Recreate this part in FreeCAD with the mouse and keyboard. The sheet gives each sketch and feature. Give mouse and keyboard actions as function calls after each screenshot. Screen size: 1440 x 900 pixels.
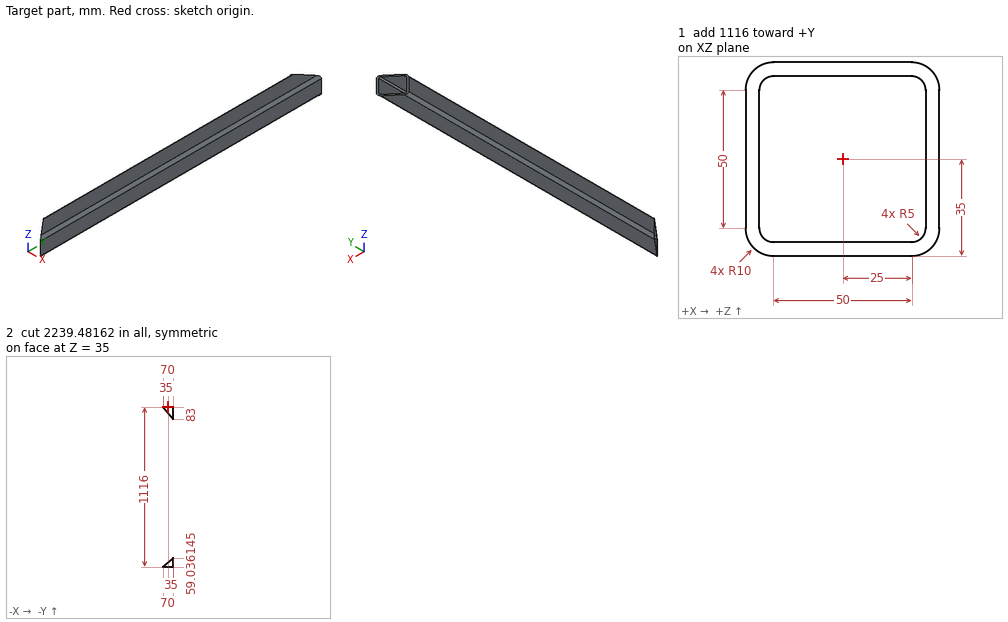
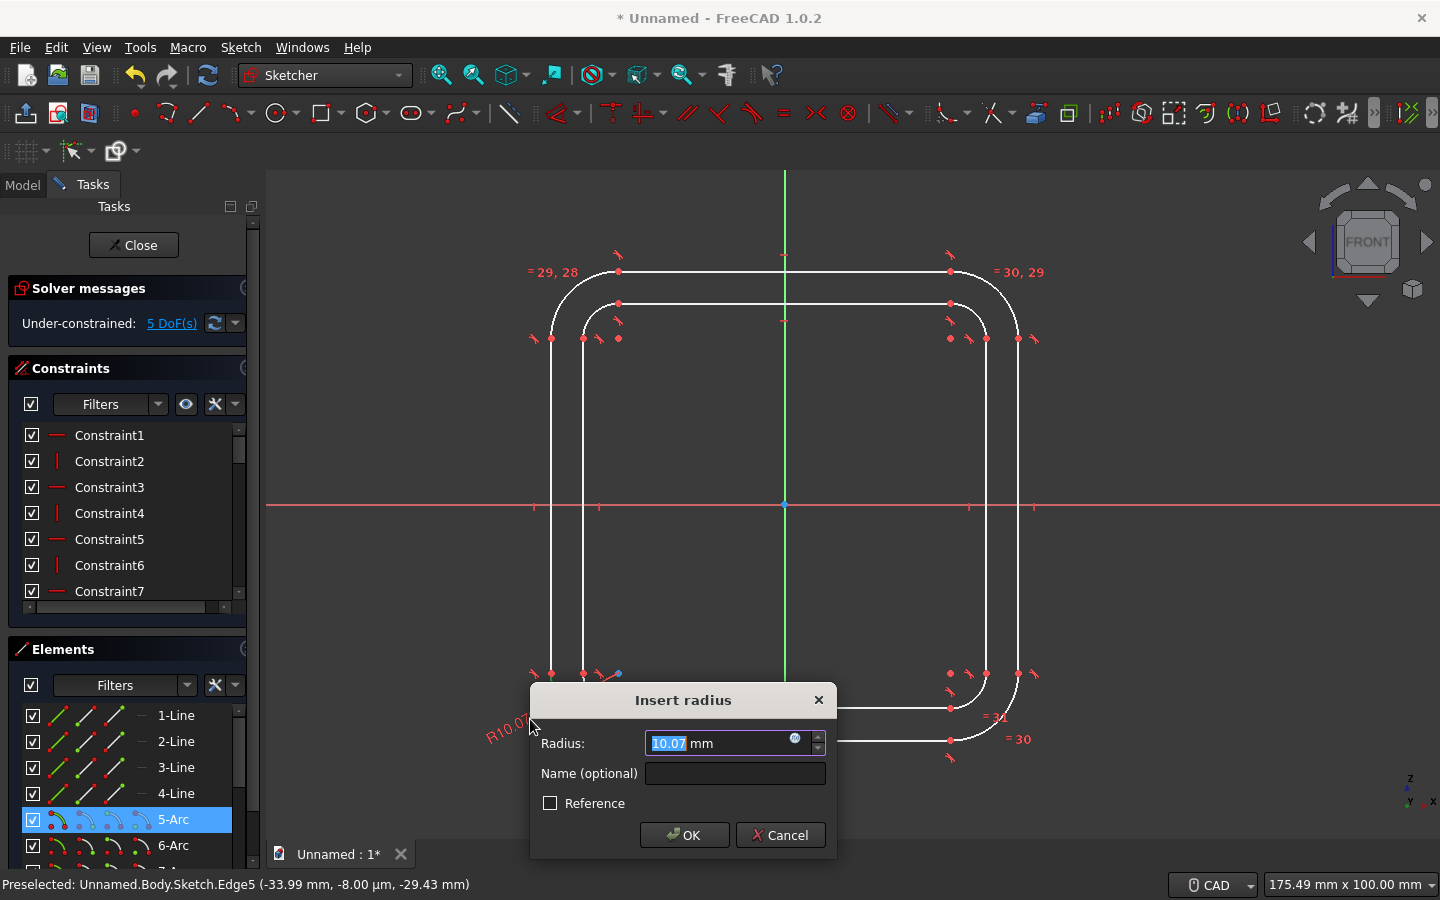
text(10)
key(Return)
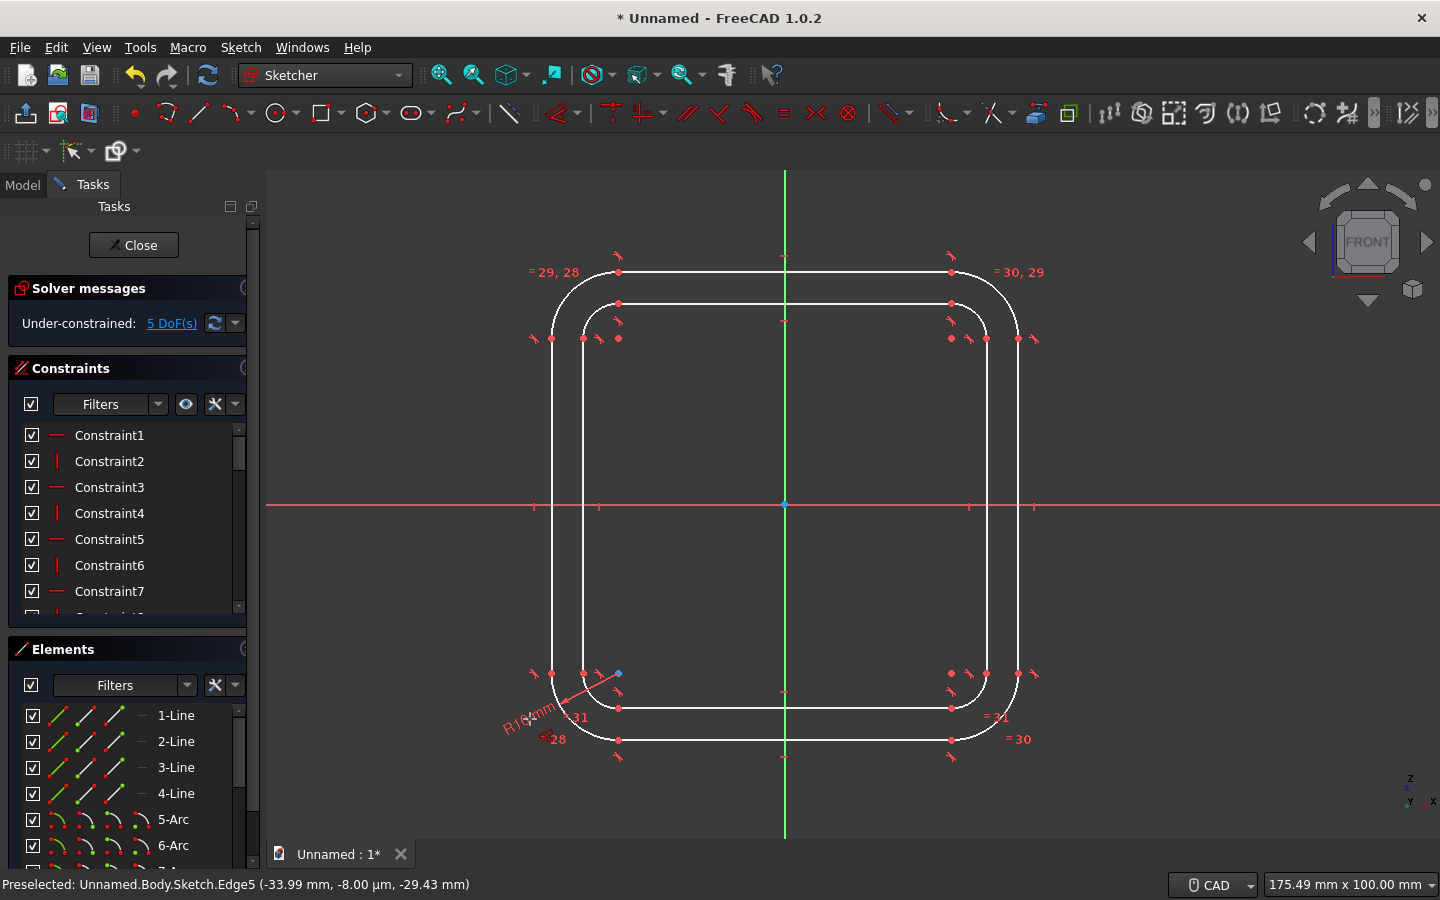
click(967, 705)
click(921, 613)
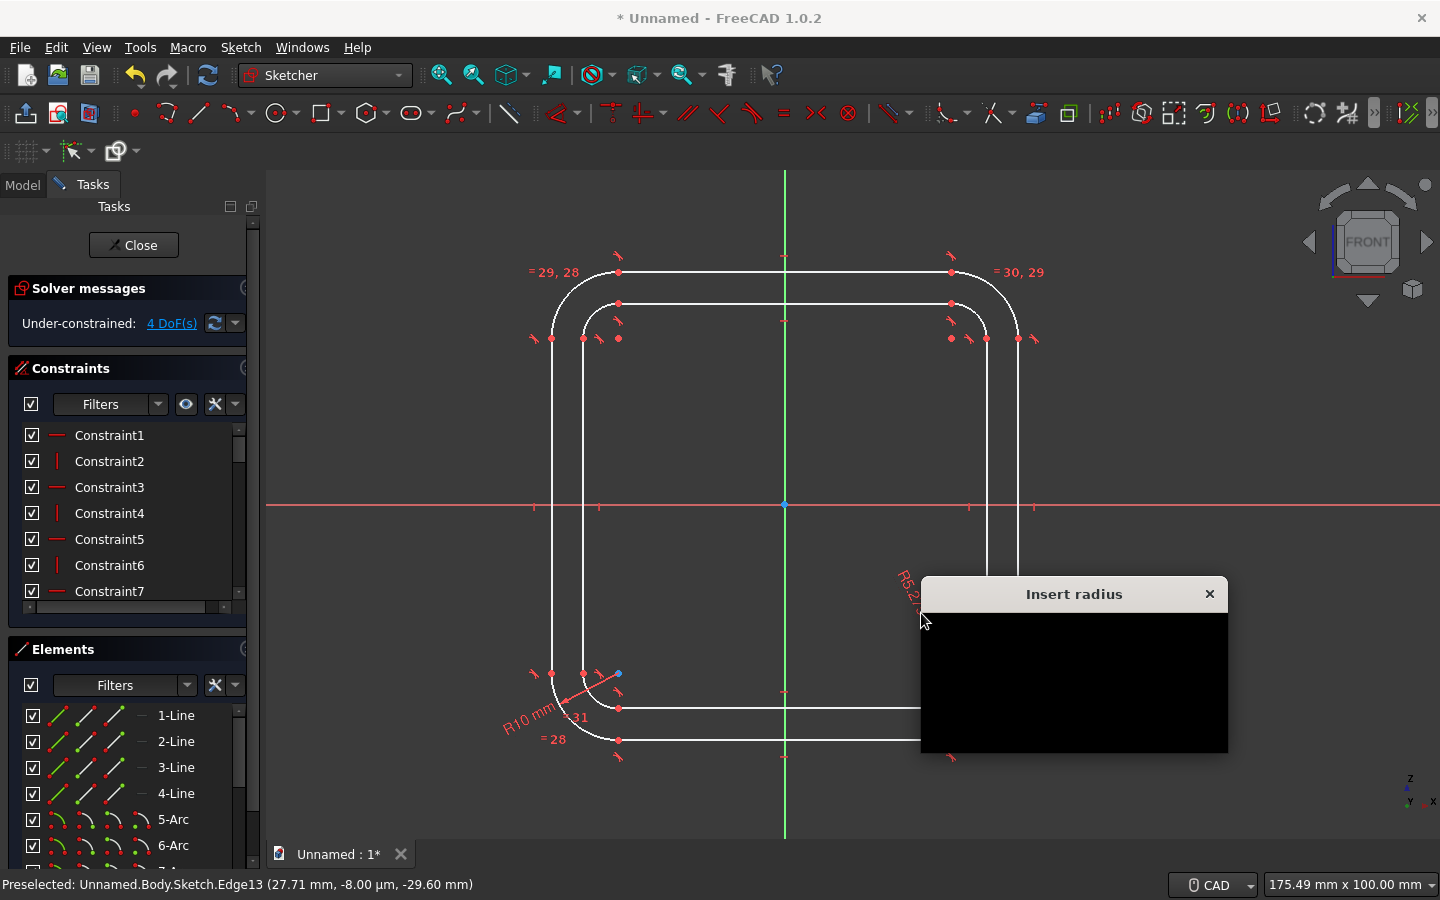
text(5)
key(Return)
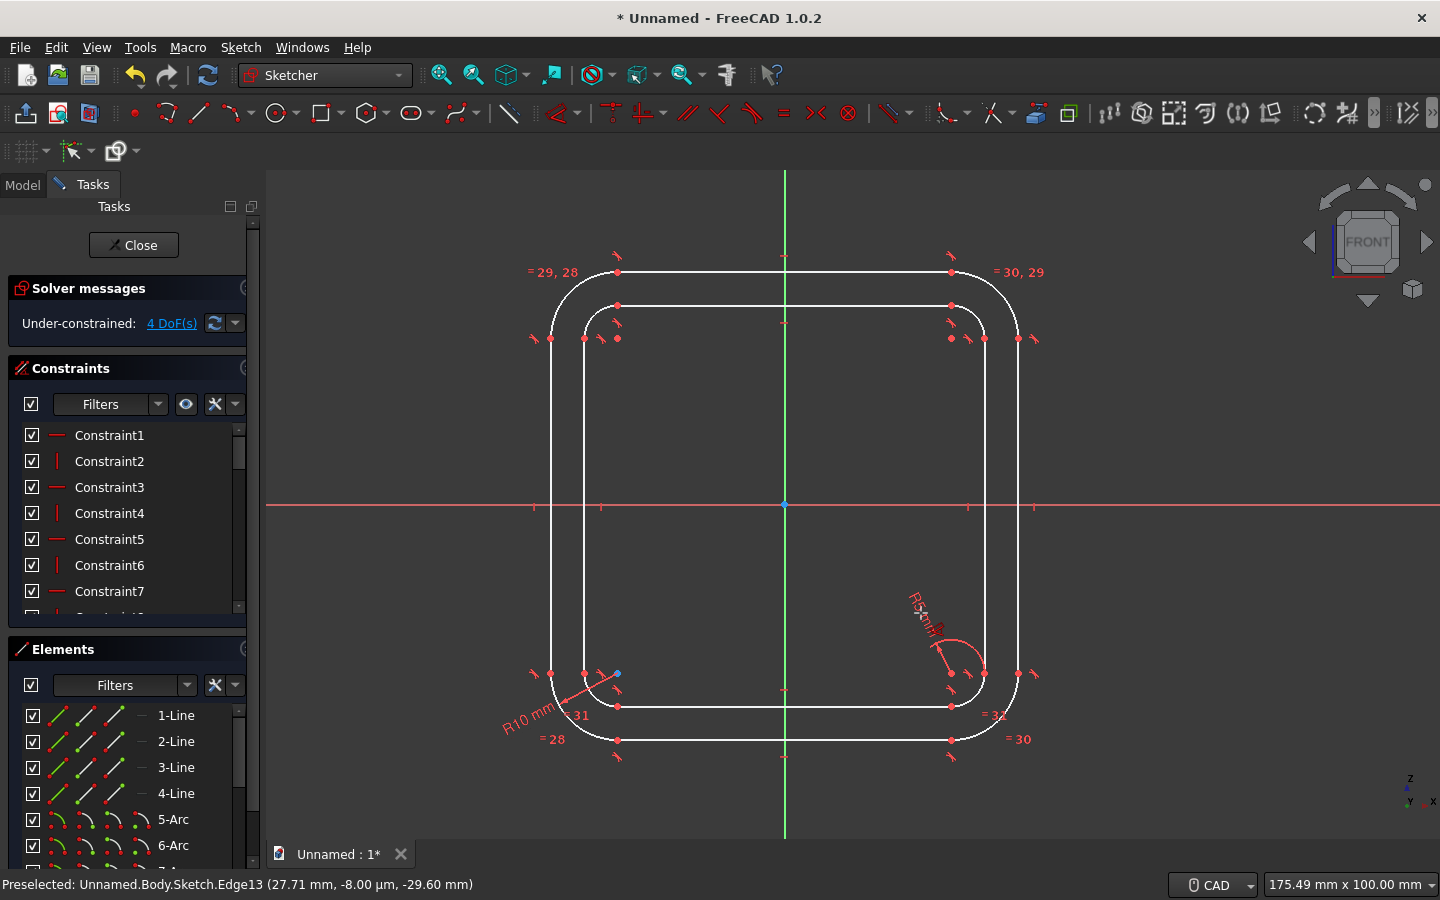
click(851, 740)
click(708, 774)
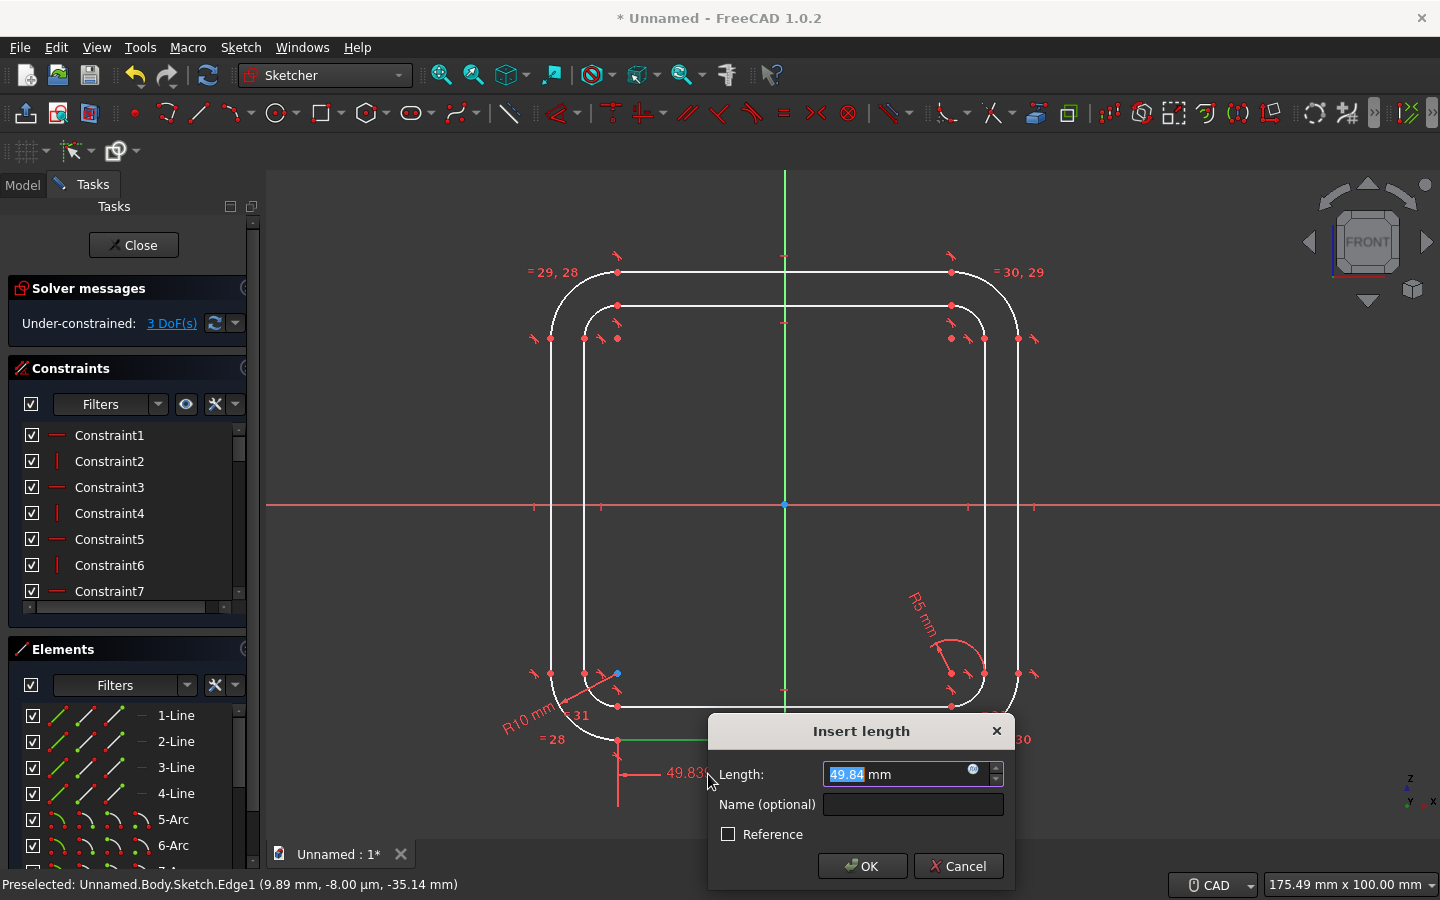
text(50)
key(Return)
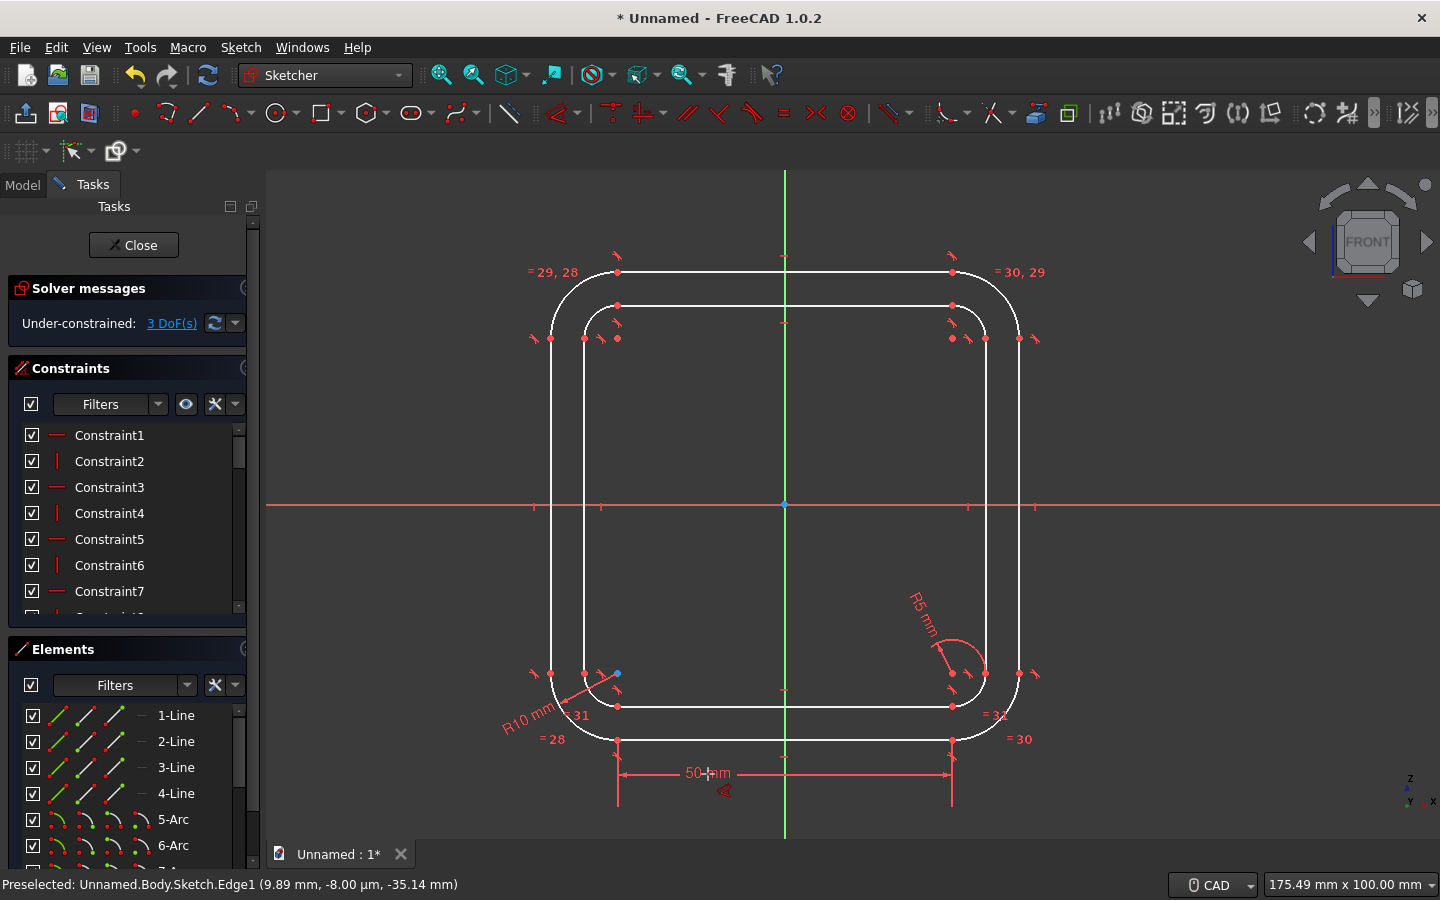
click(551, 573)
click(517, 429)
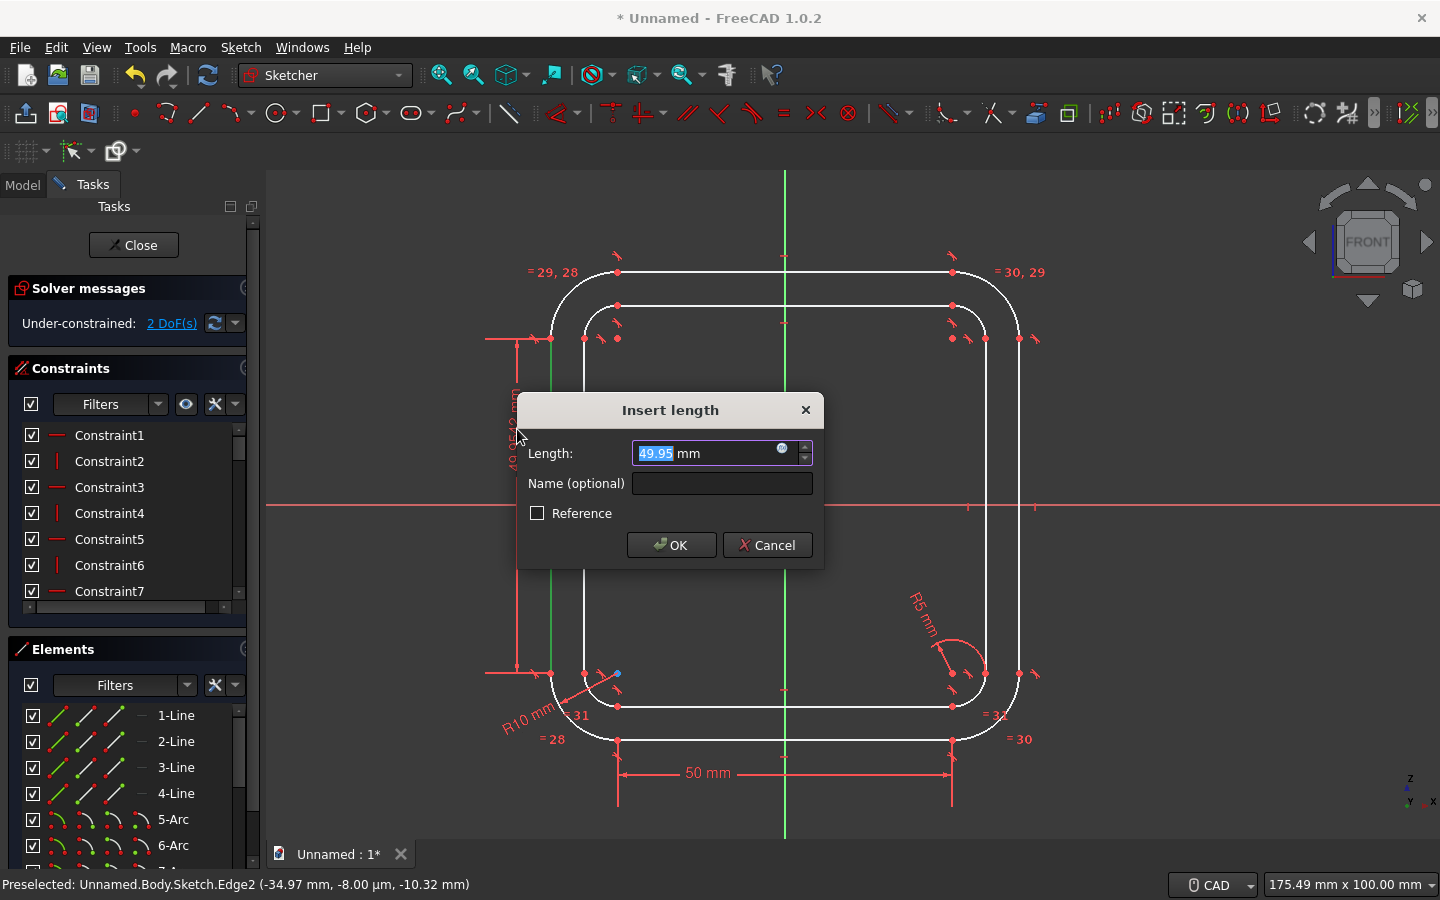
text(50)
key(Return)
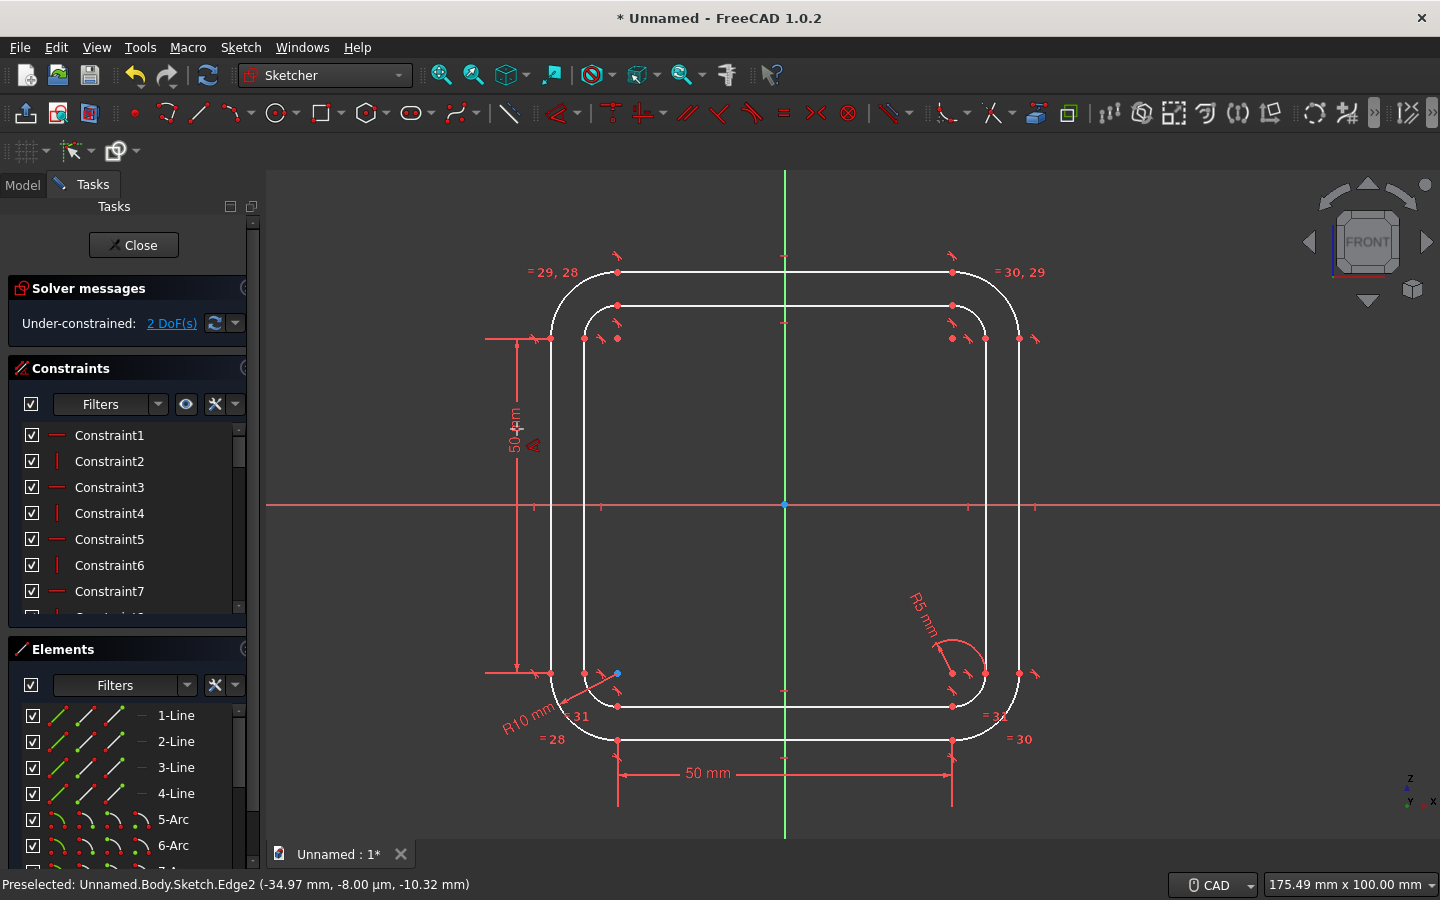
click(952, 740)
click(869, 774)